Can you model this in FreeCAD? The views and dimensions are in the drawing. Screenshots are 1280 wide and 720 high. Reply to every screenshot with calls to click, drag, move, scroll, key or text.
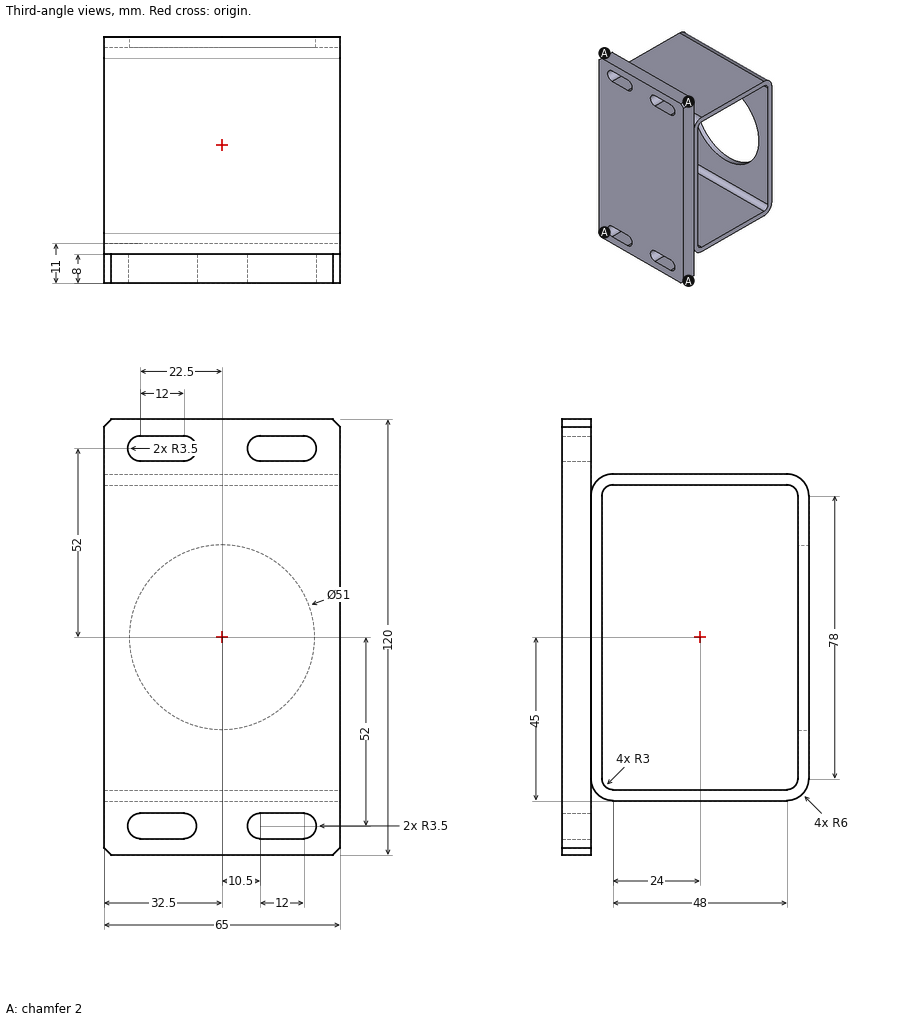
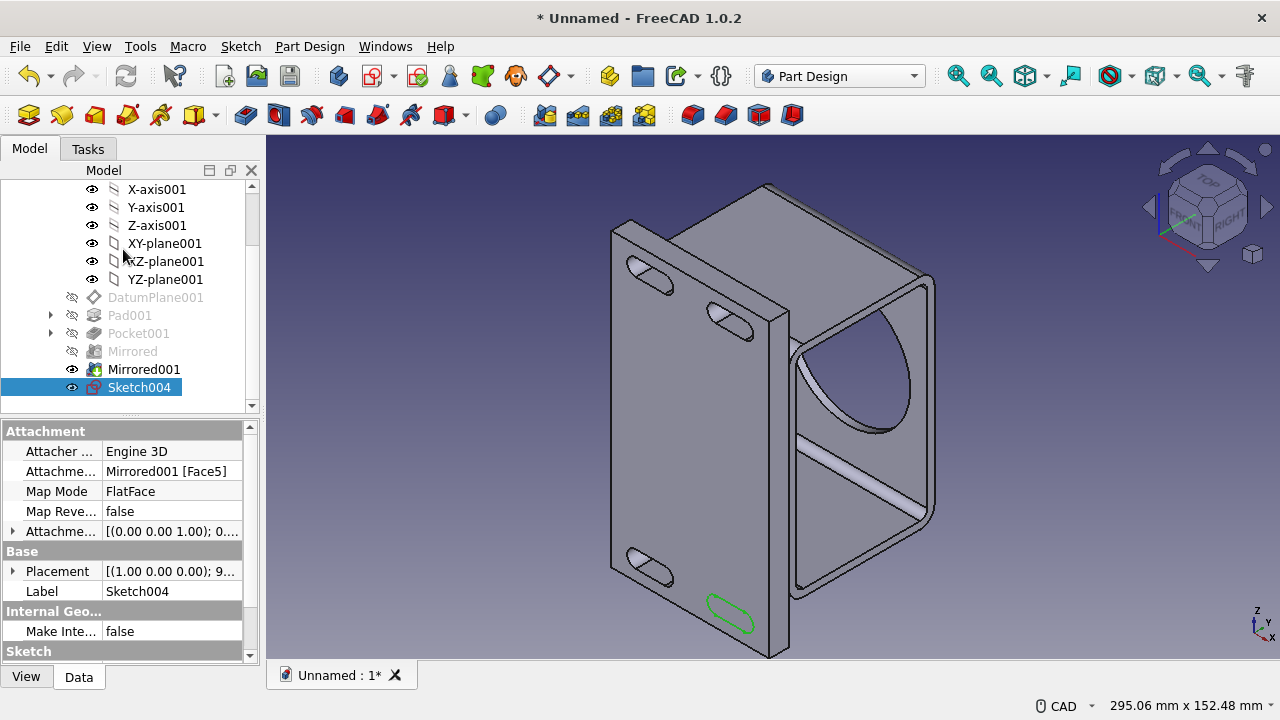
click(246, 116)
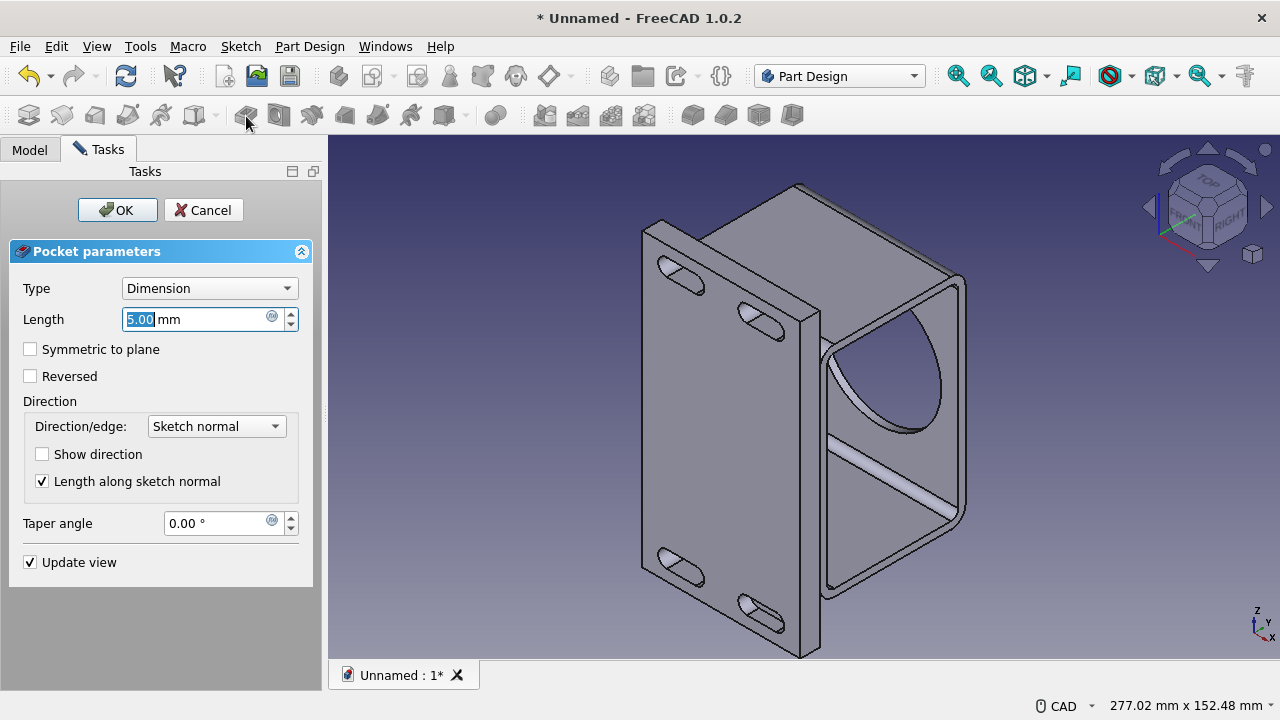
text(11)
key(Tab)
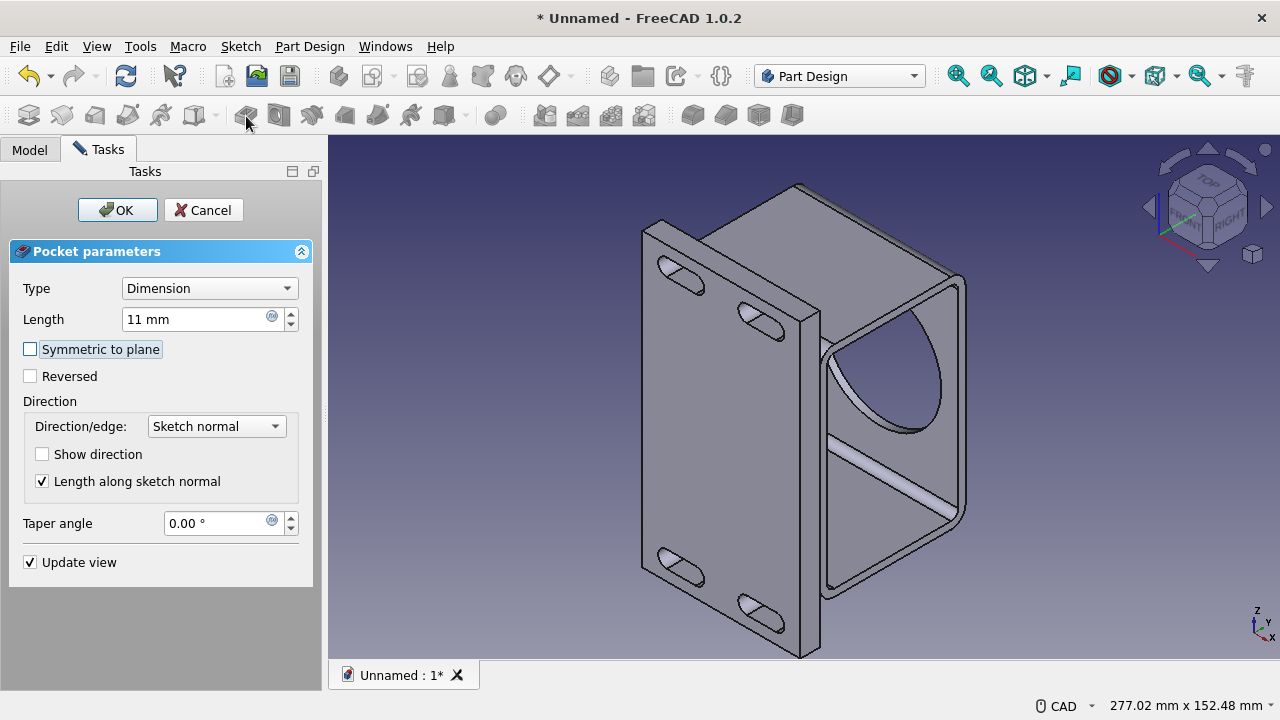
click(118, 210)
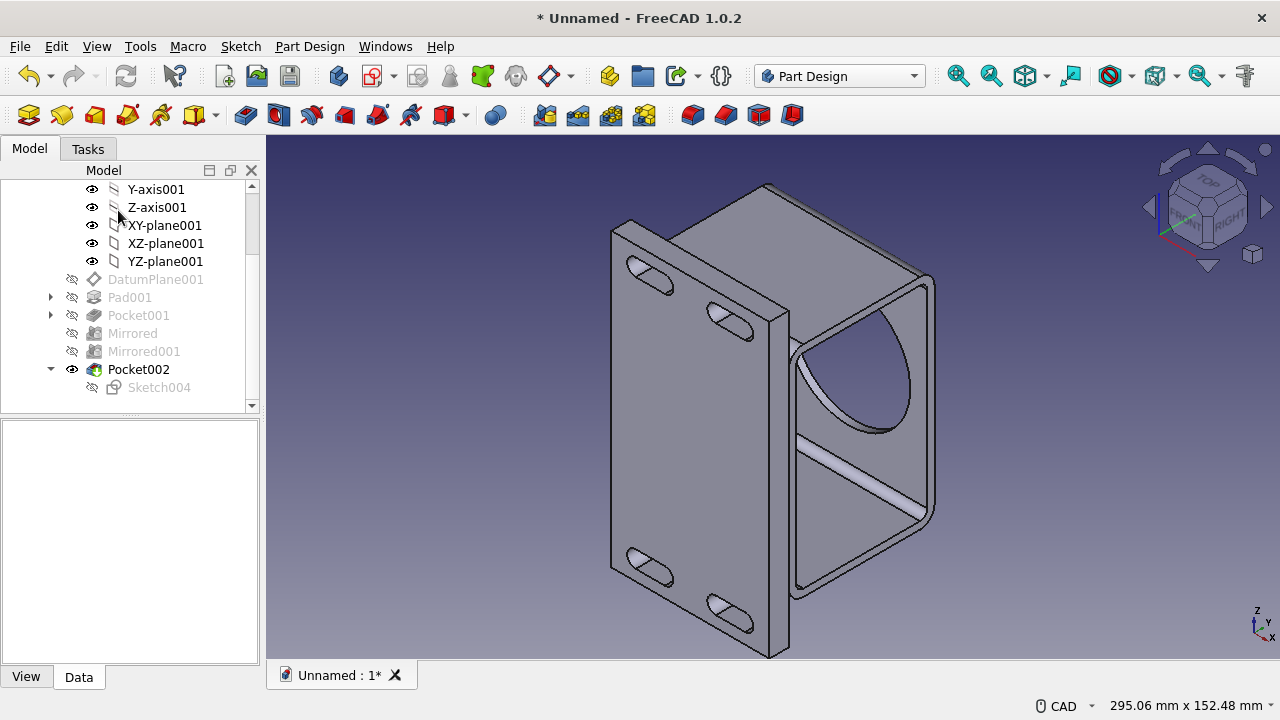
click(779, 315)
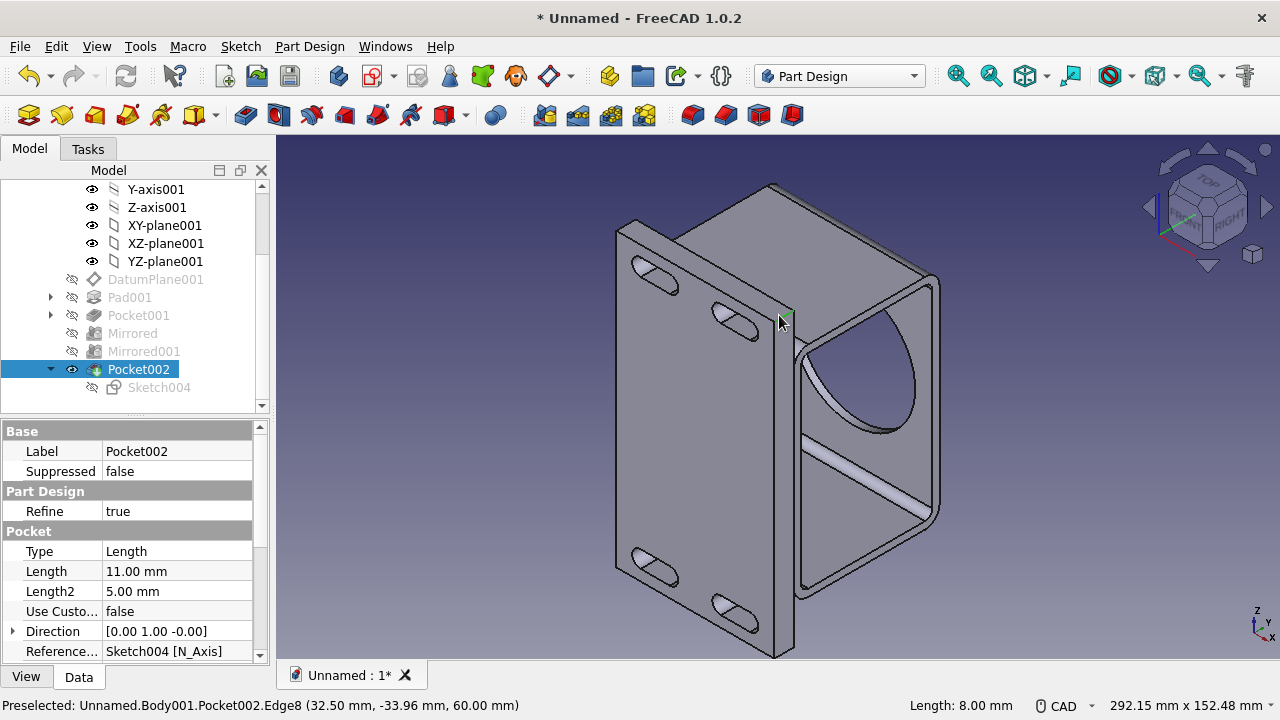
key(2)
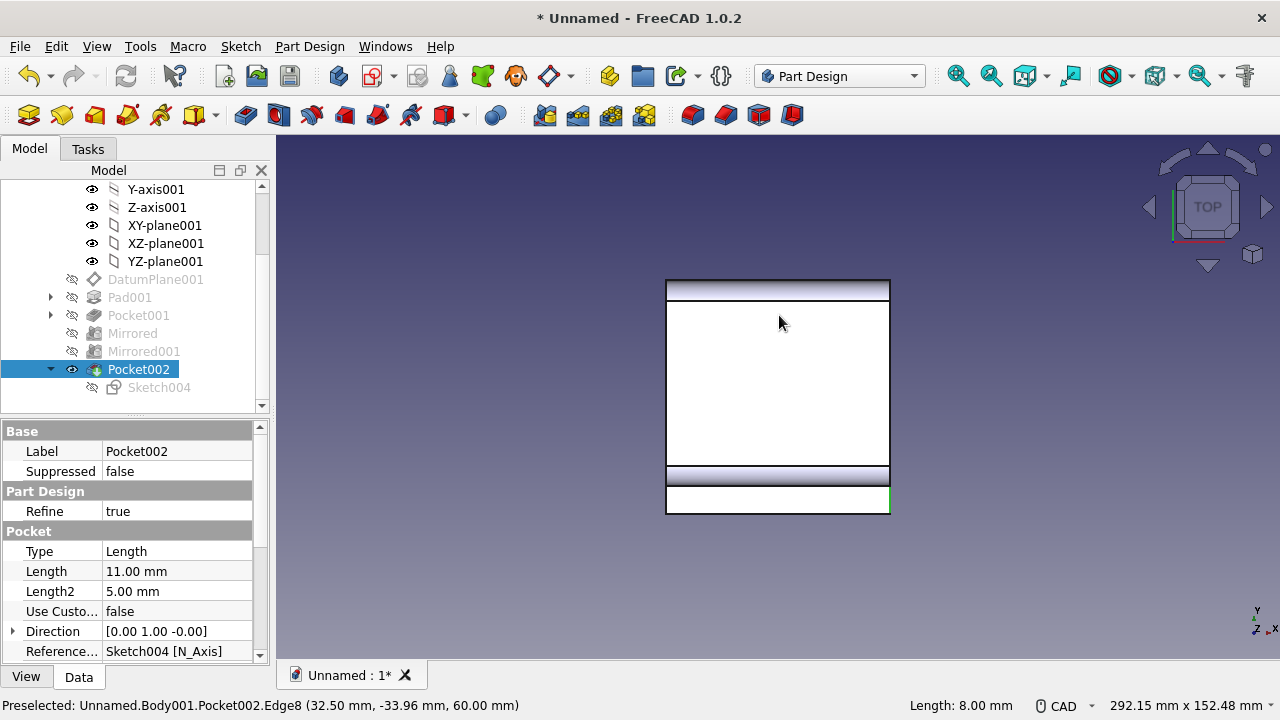
click(959, 76)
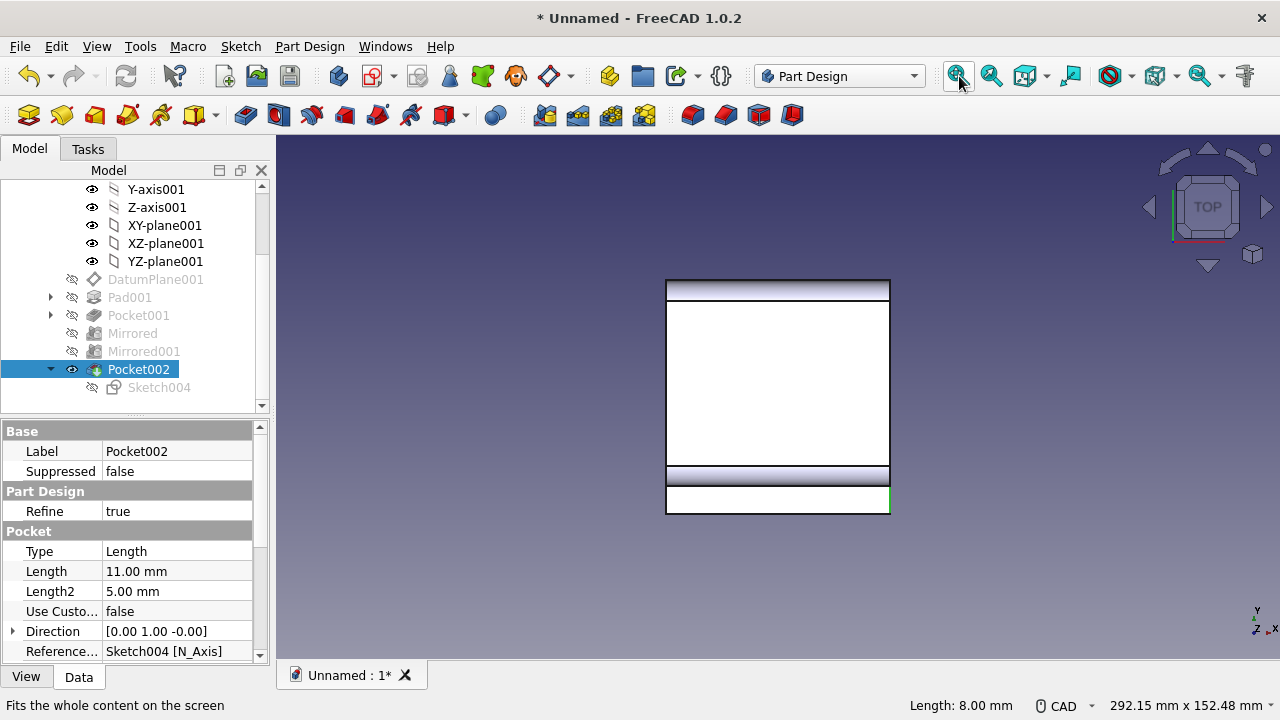
click(666, 499, ctrl)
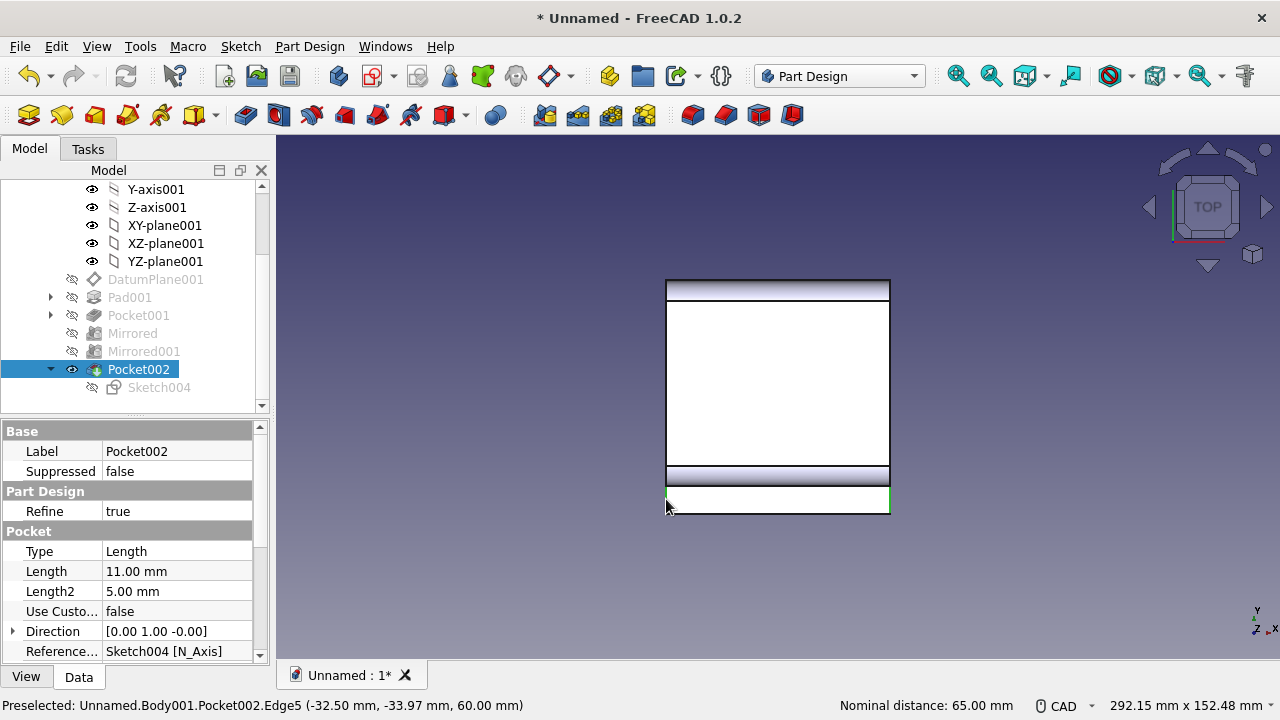
key(0)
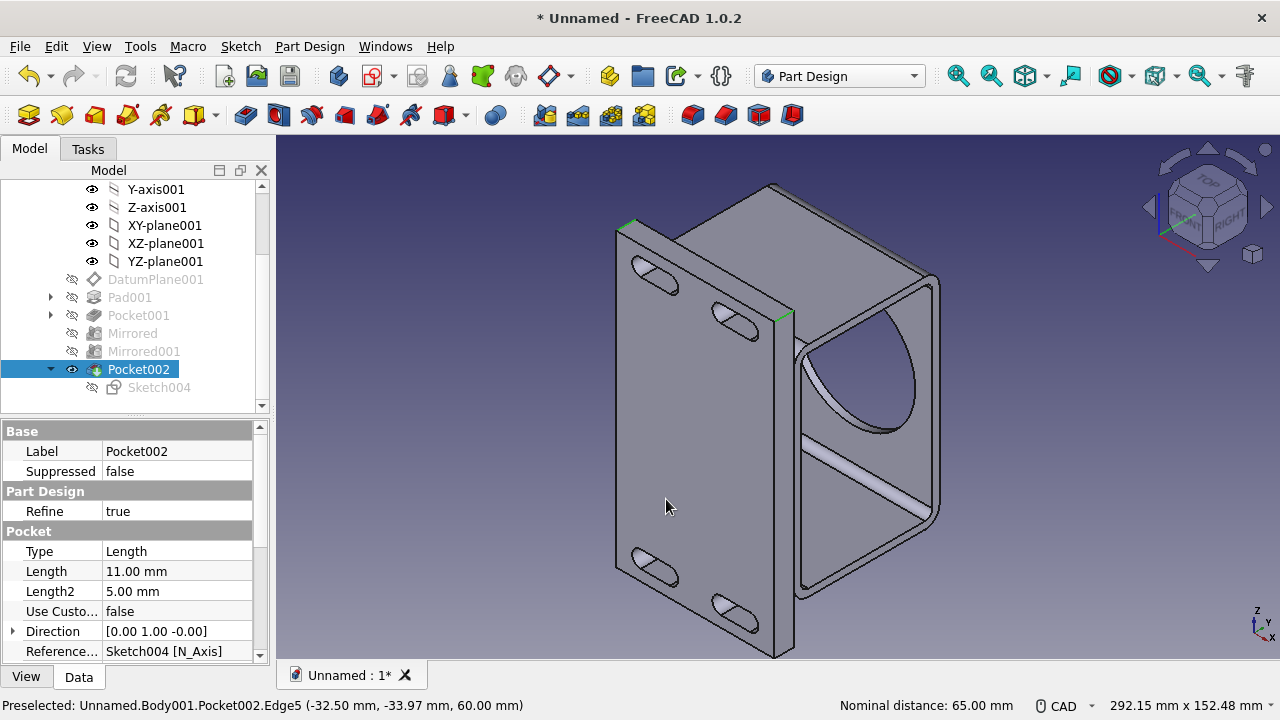
key(1)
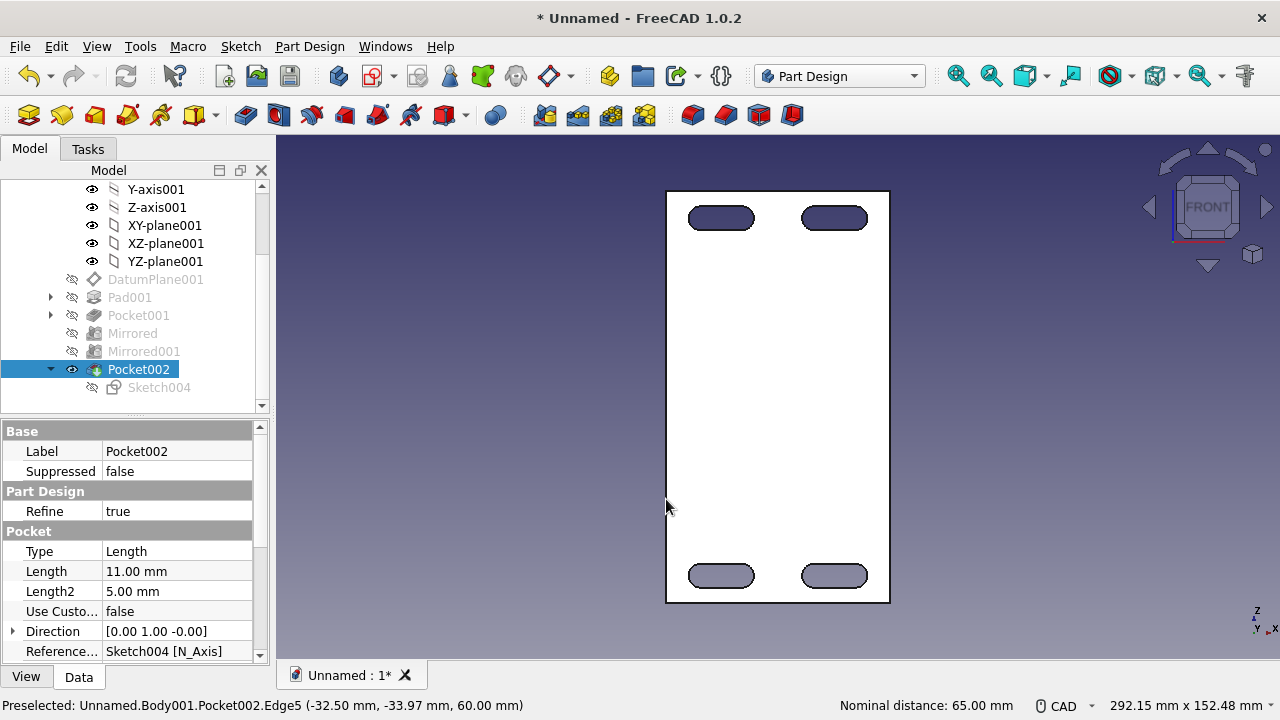
key(3)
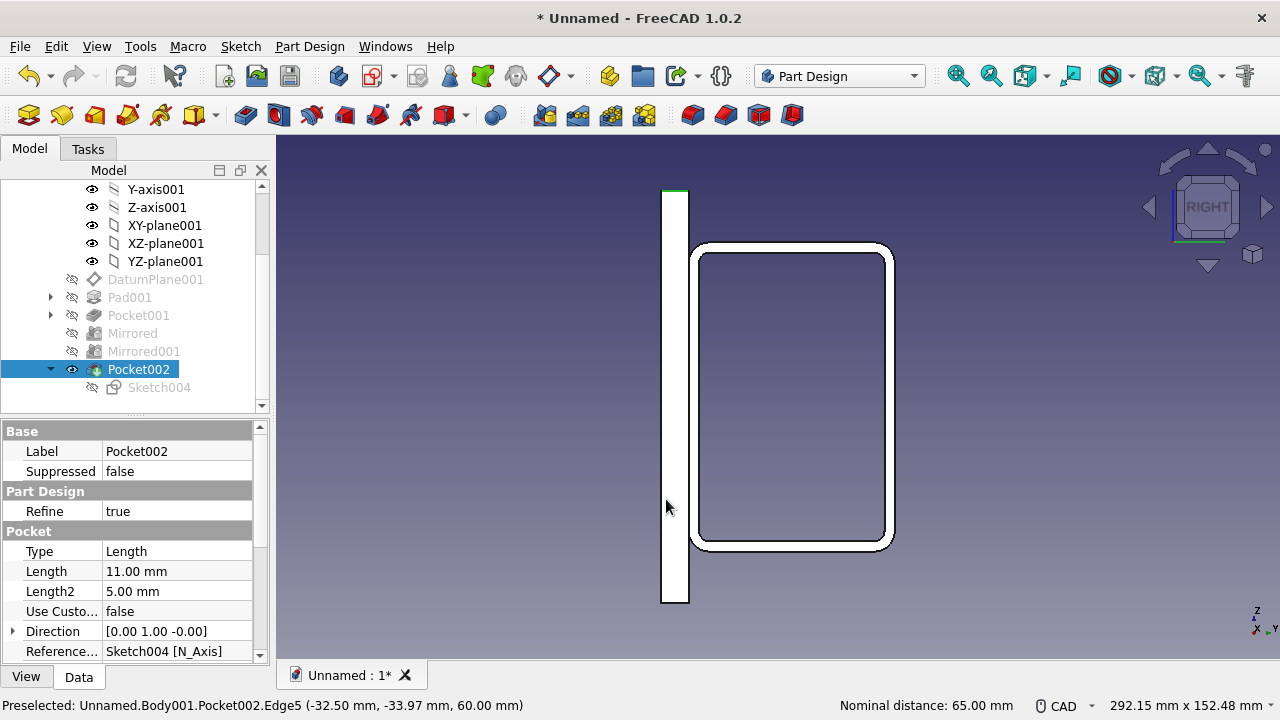
click(675, 602, ctrl)